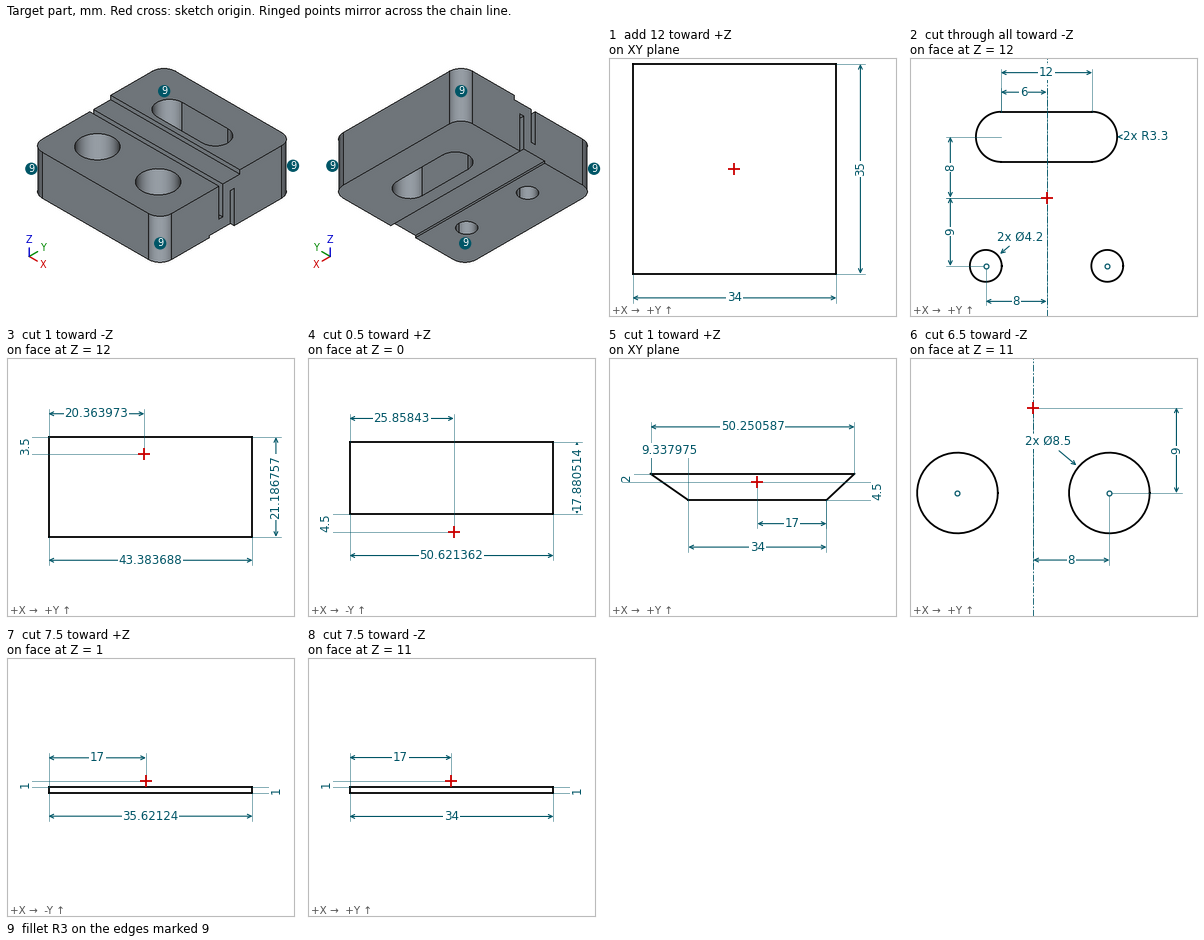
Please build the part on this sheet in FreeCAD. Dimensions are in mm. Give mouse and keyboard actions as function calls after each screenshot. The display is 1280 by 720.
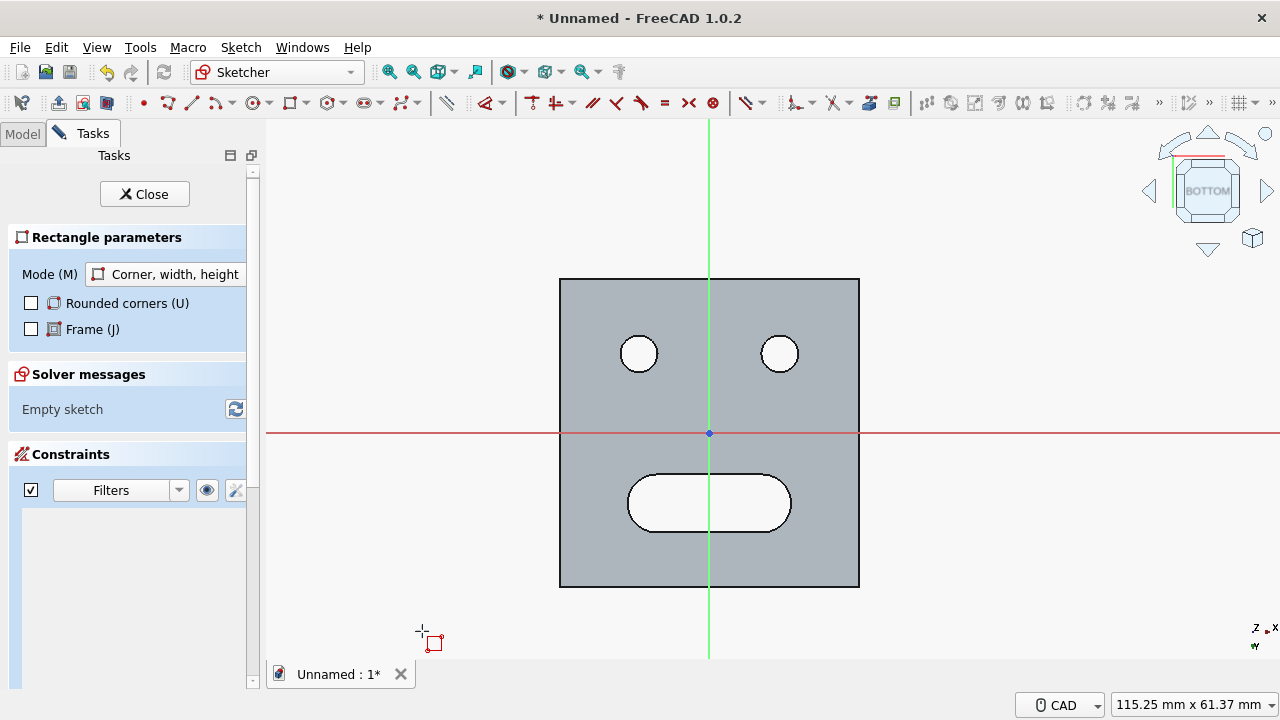
click(482, 236)
move(927, 393)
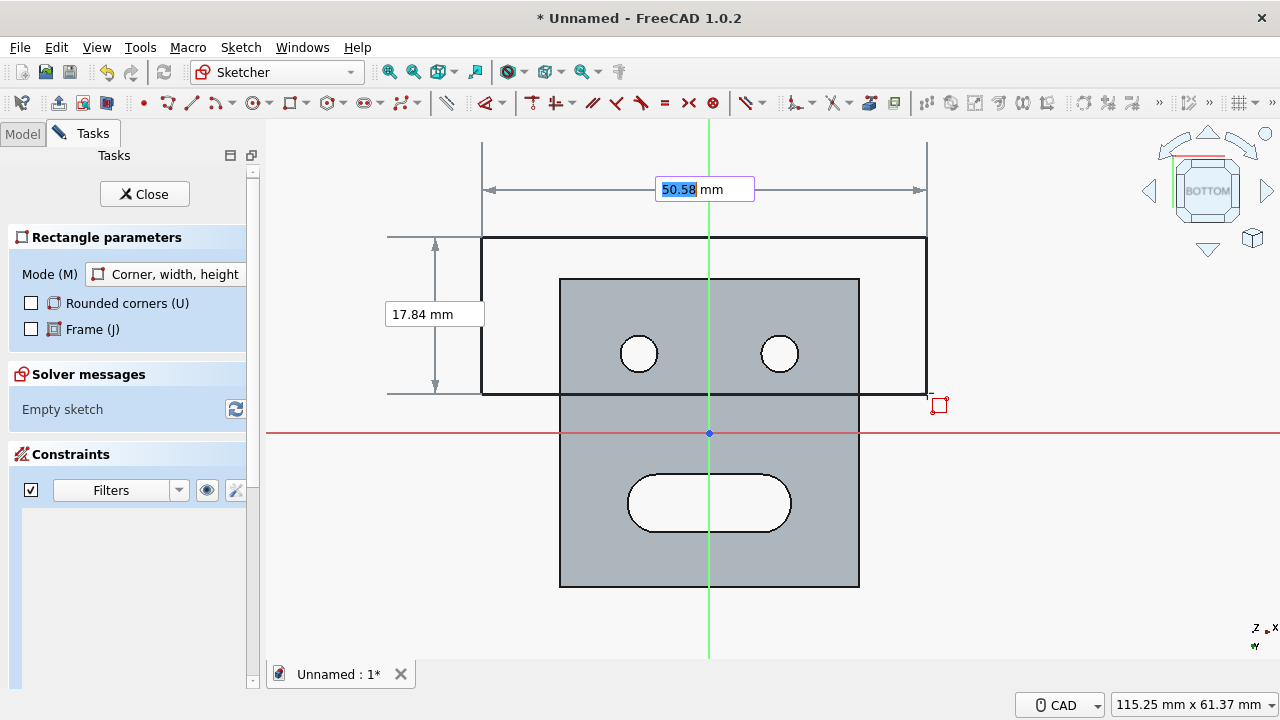
text(50.621362)
key(Tab)
text(17.880514)
key(Return)
key(Escape)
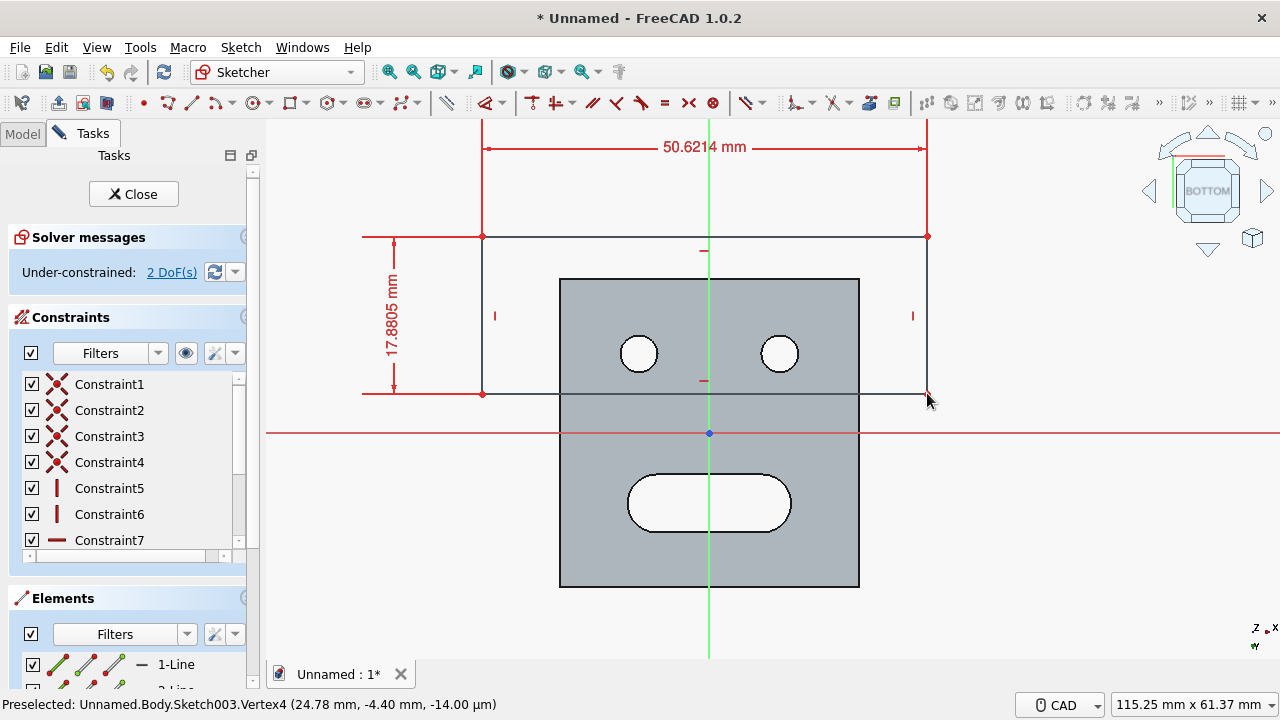
click(486, 104)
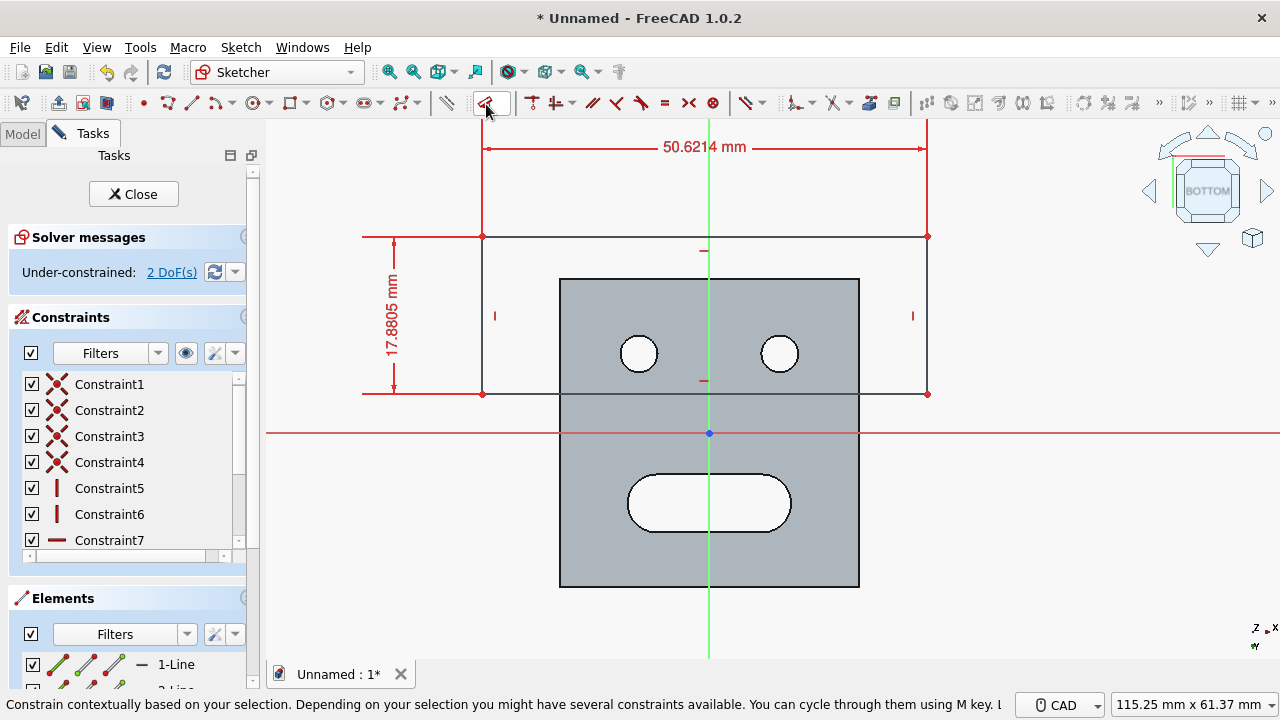
click(482, 394)
click(448, 414)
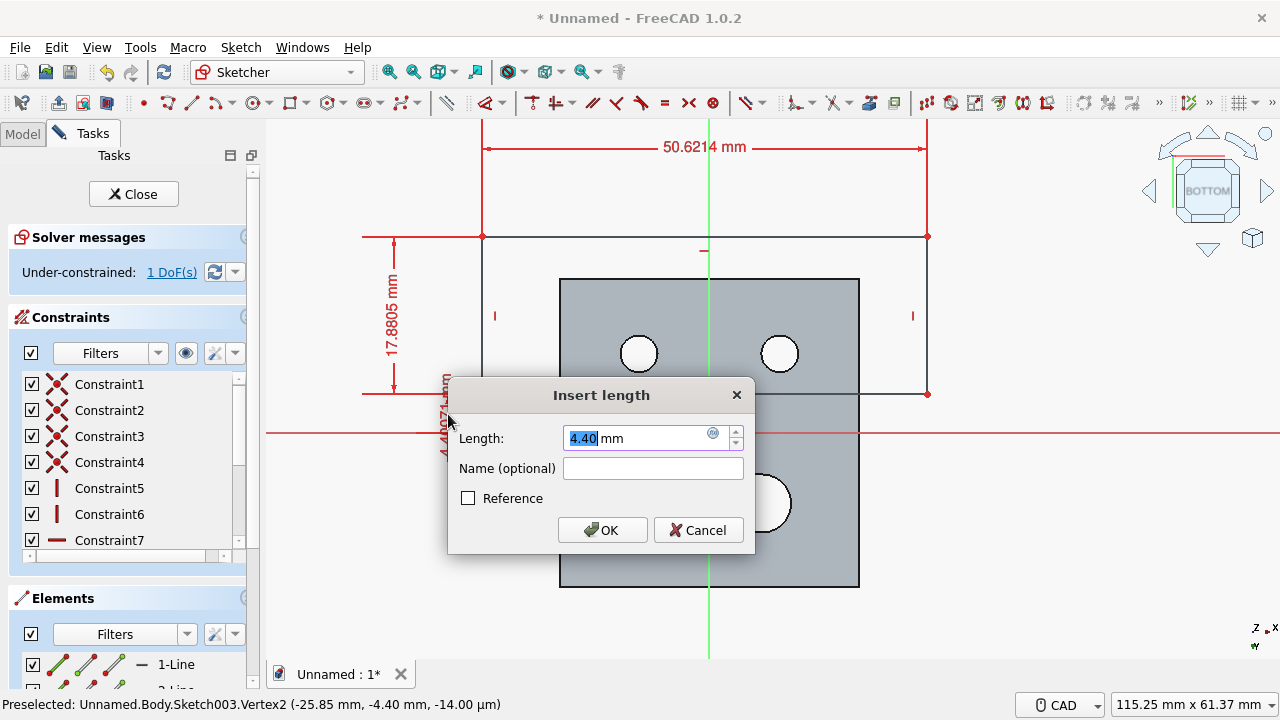
text(4.5)
key(Return)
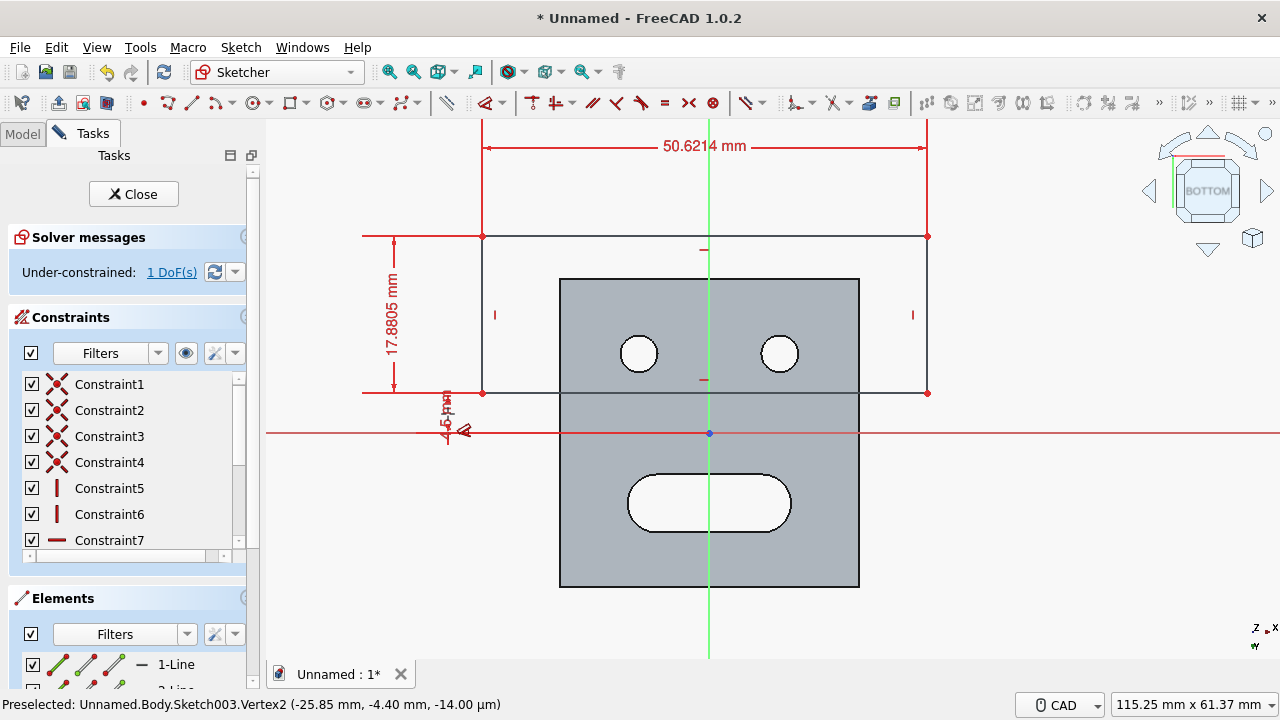
click(482, 236)
click(596, 202)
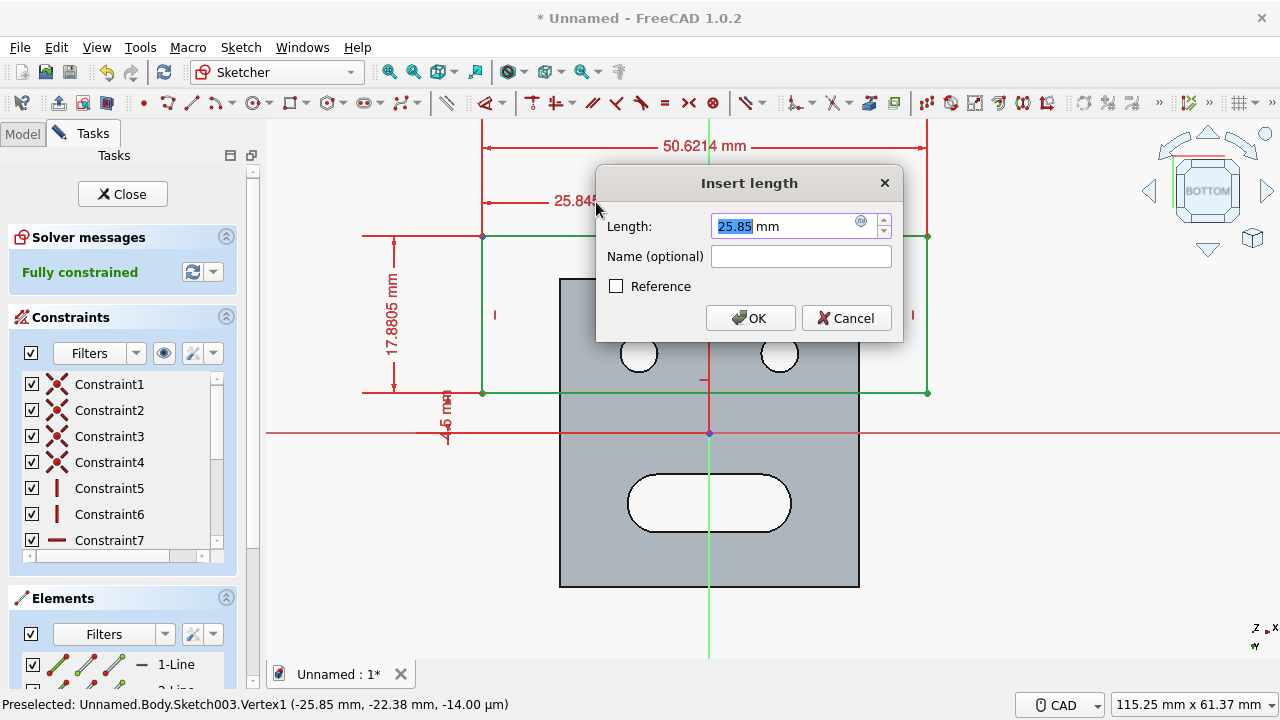
text(25.85843)
key(Return)
key(Escape)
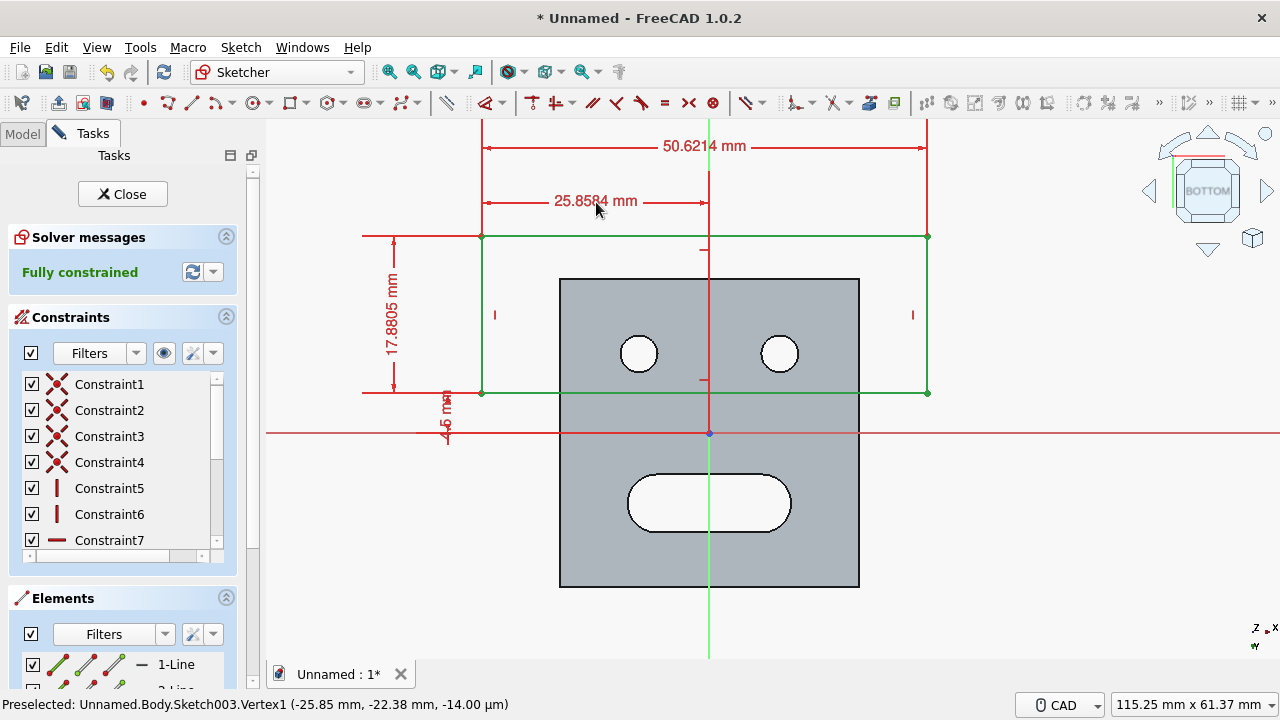
click(123, 194)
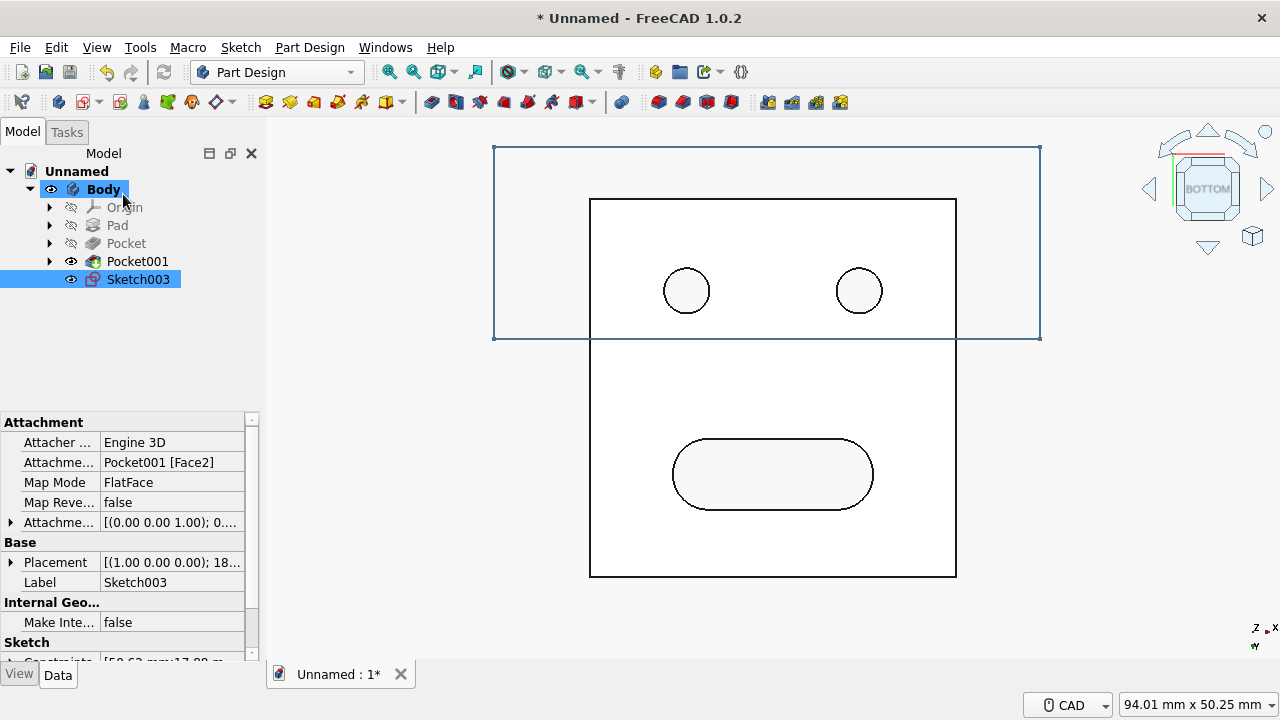
click(432, 102)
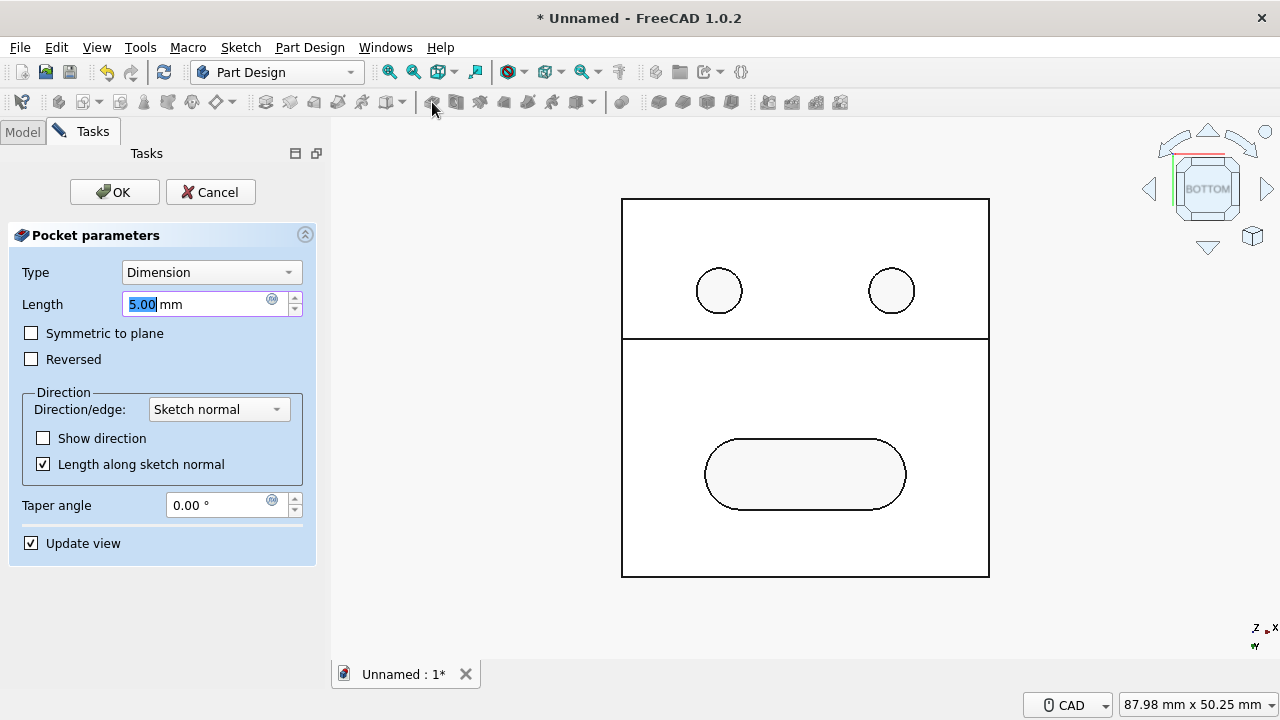
text(0.5)
key(Tab)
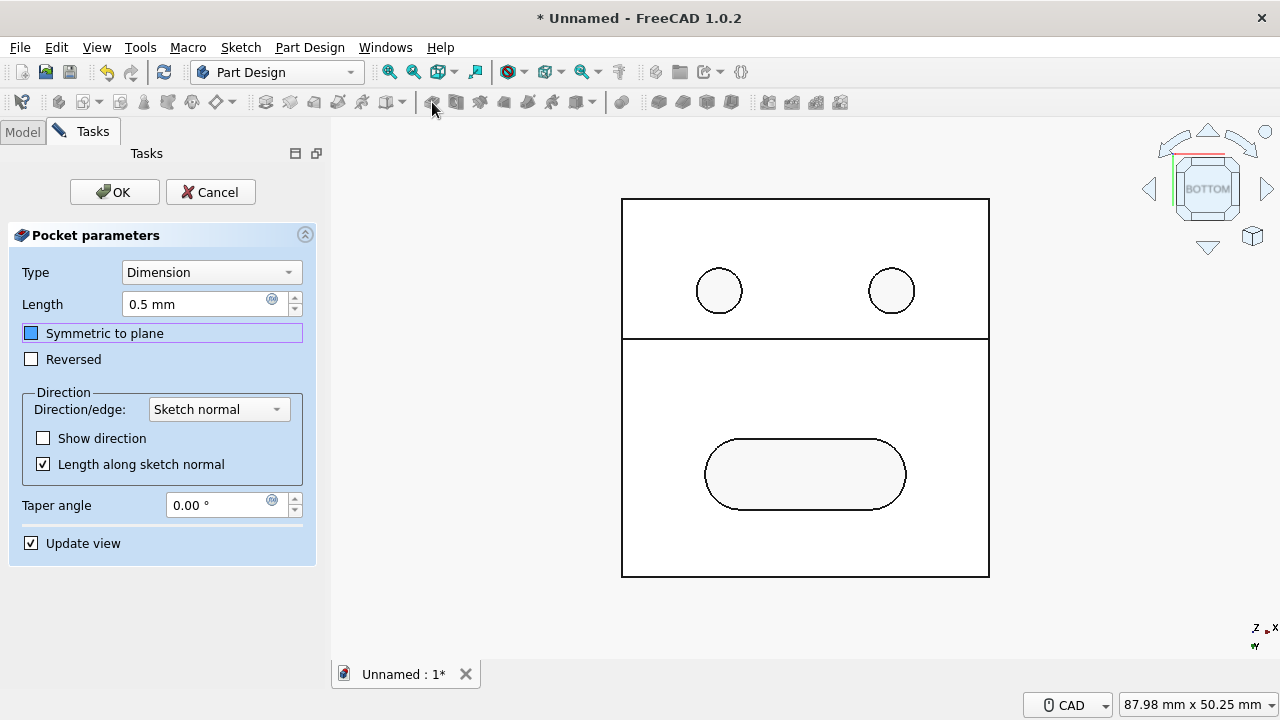
click(115, 192)